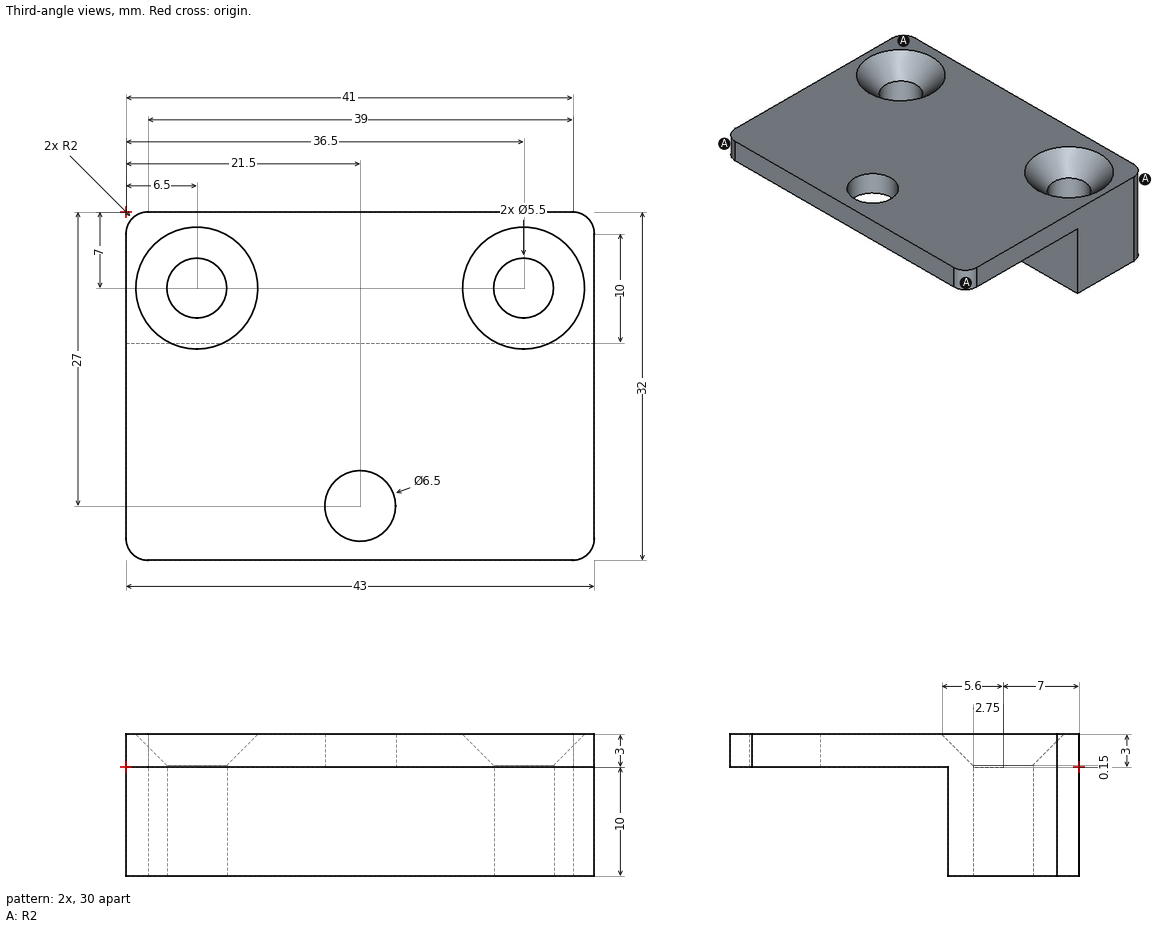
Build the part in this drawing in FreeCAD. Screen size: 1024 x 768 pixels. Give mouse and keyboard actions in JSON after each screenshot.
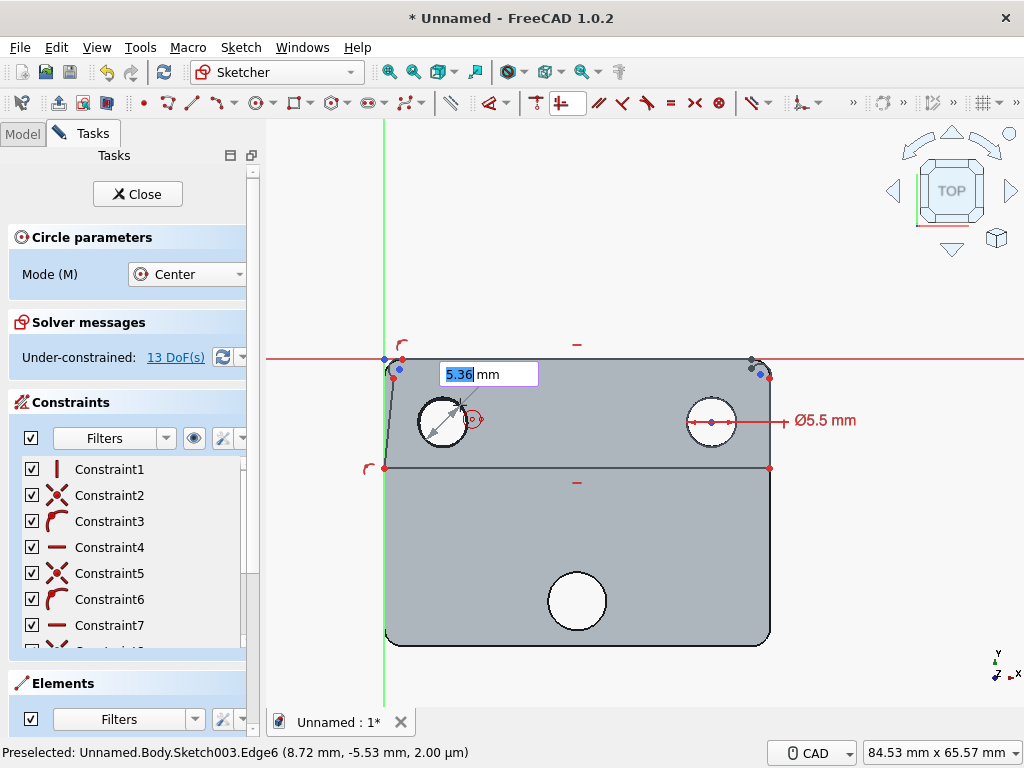
{"action": "type", "text": "5.5"}
{"action": "key", "text": "Return"}
{"action": "key", "text": "Escape"}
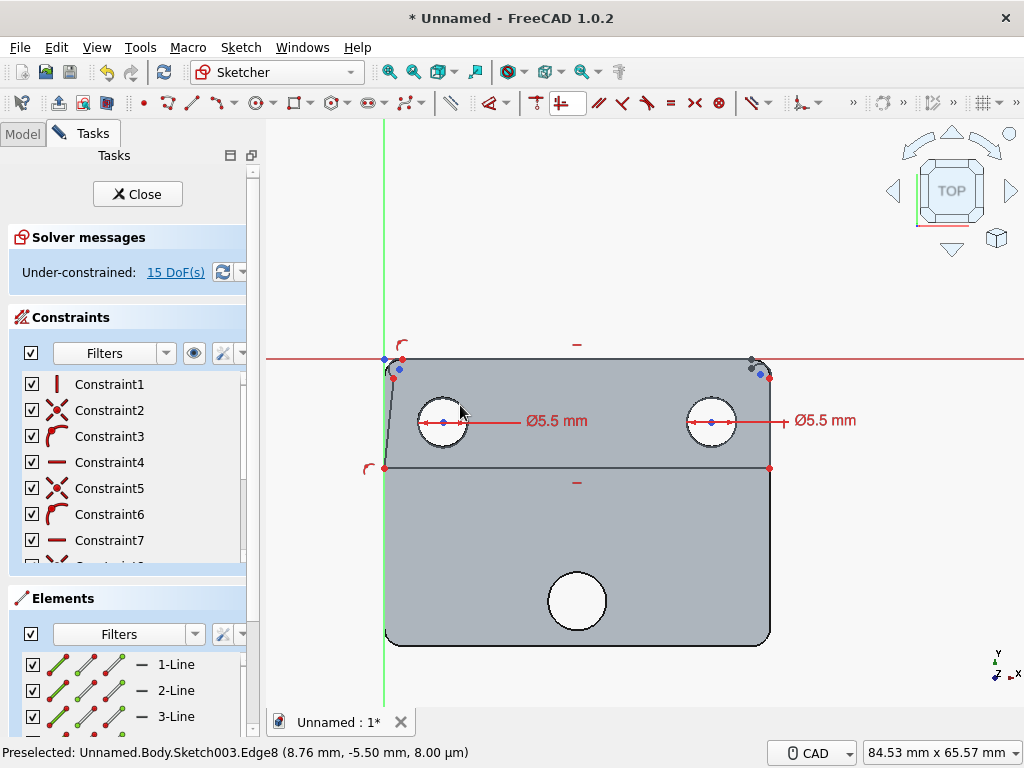
{"action": "left_click", "coordinate": [770, 405]}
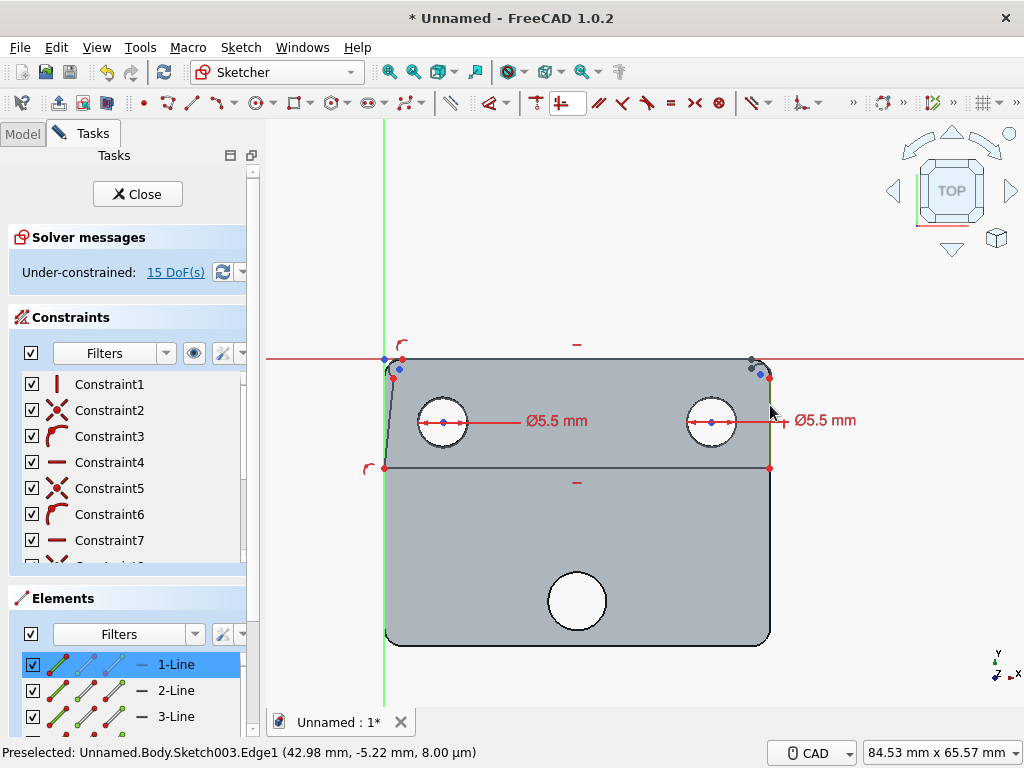
{"action": "scroll", "coordinate": [770, 369], "scroll_direction": "up", "scroll_amount": 3}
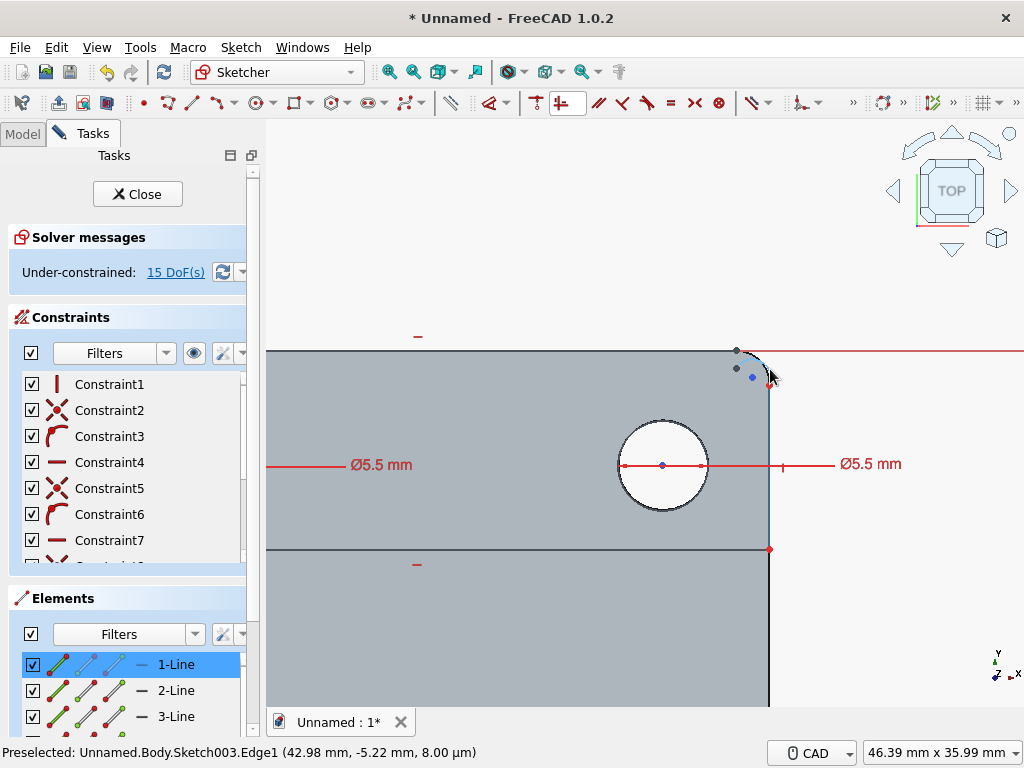
{"action": "left_click", "coordinate": [769, 369]}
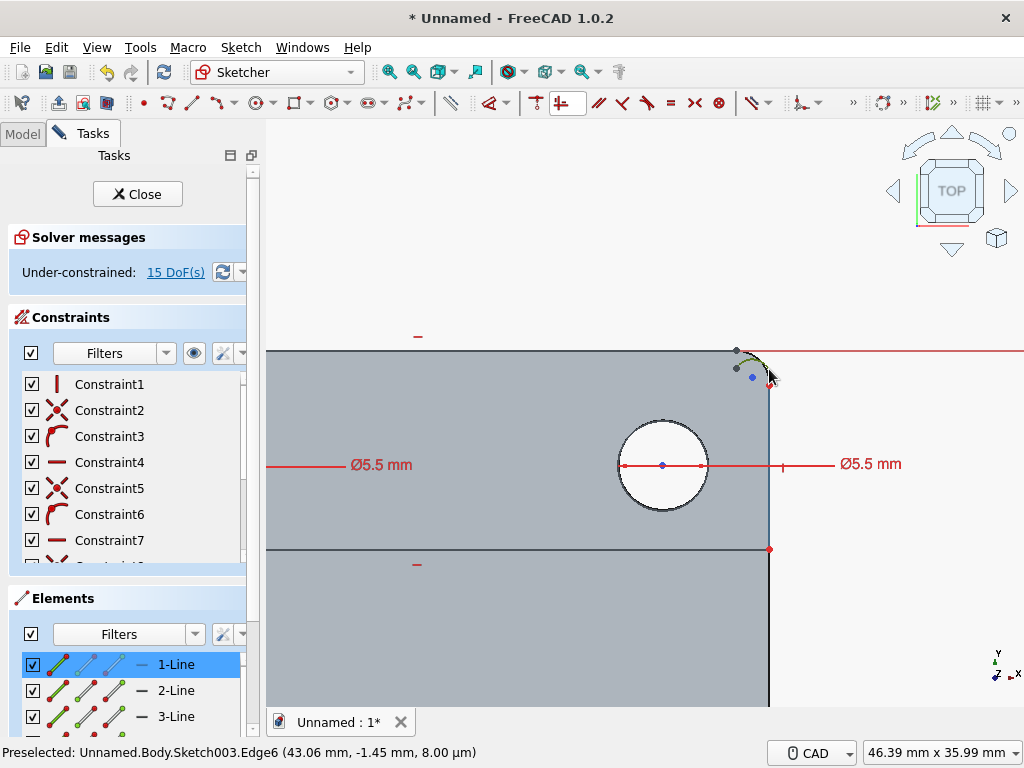
{"action": "key", "text": "t"}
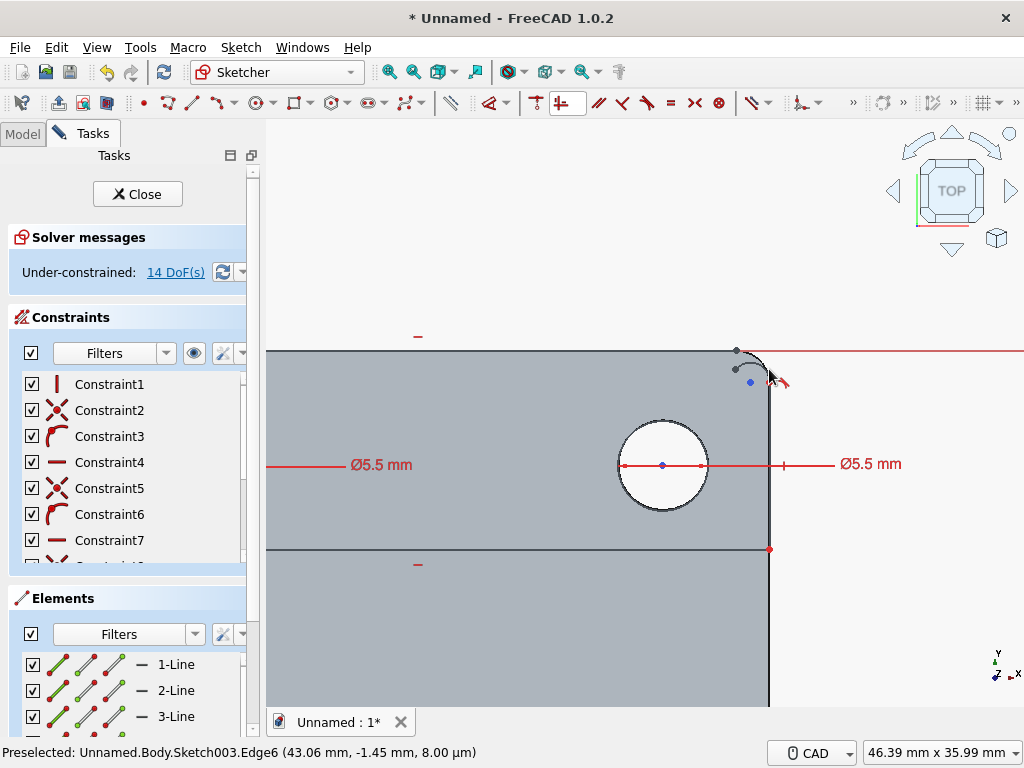
{"action": "scroll", "coordinate": [769, 369], "scroll_direction": "down", "scroll_amount": 3}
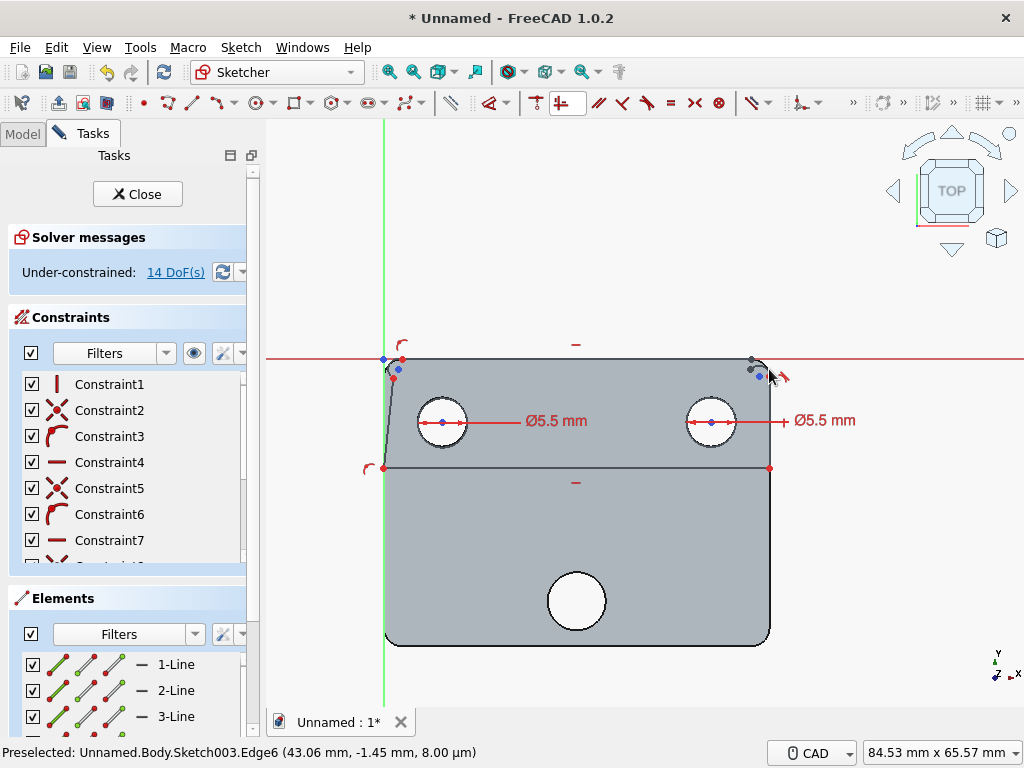
{"action": "scroll", "coordinate": [391, 405], "scroll_direction": "up", "scroll_amount": 4}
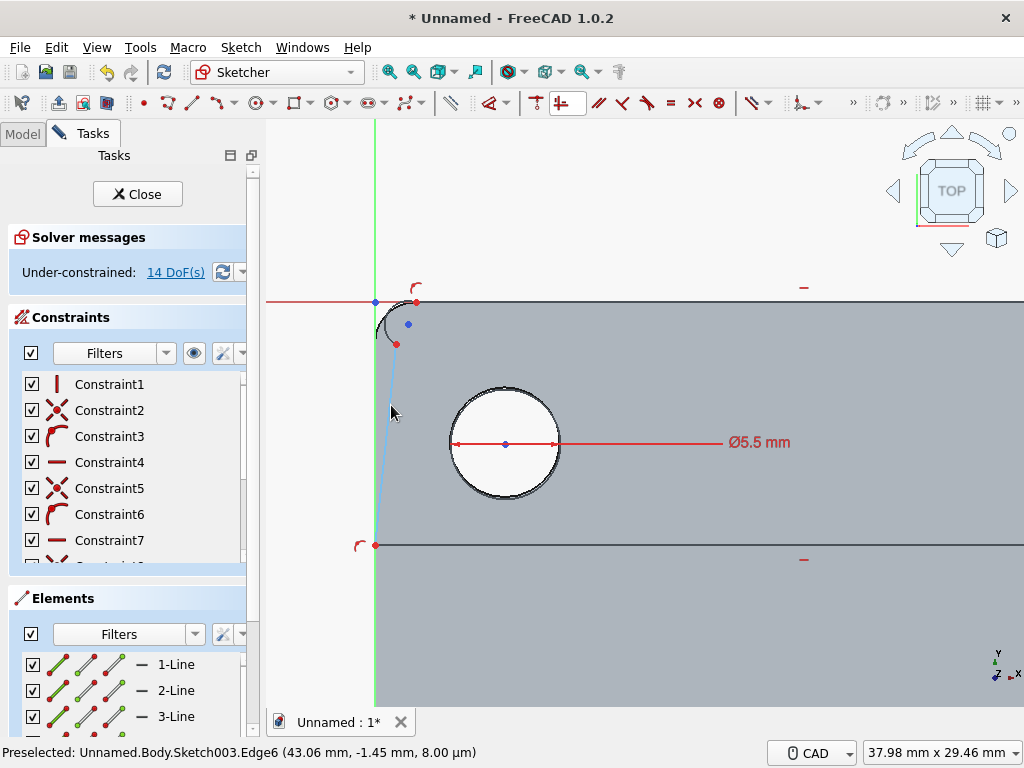
{"action": "left_click", "coordinate": [390, 405]}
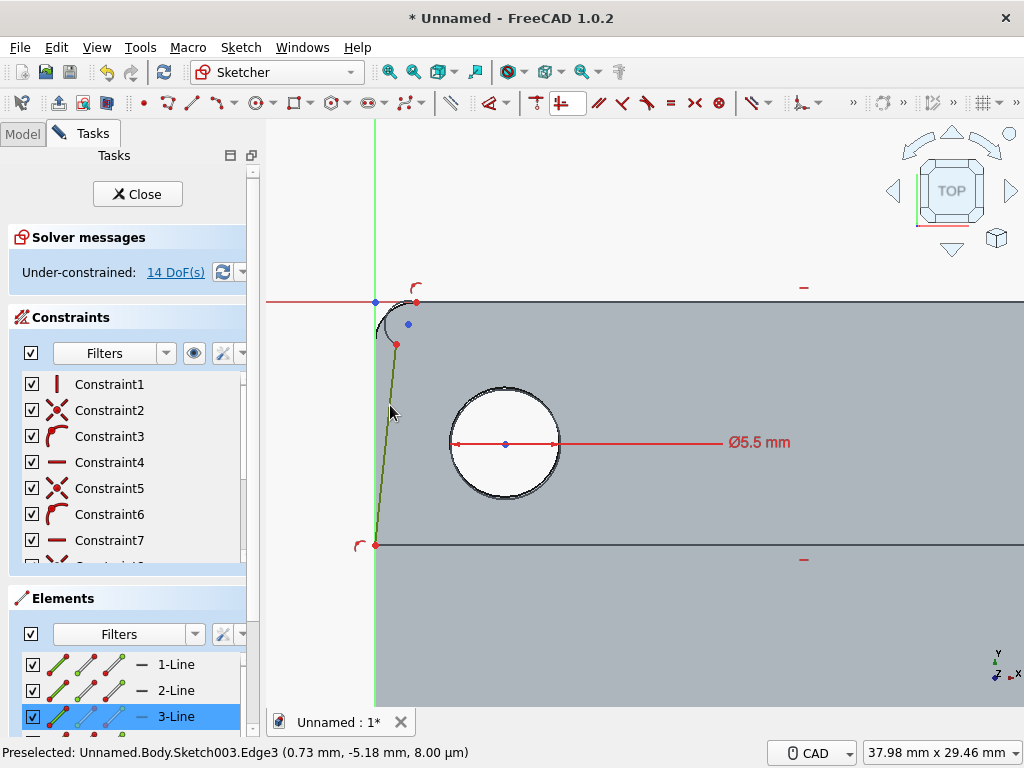
{"action": "left_click", "coordinate": [396, 305]}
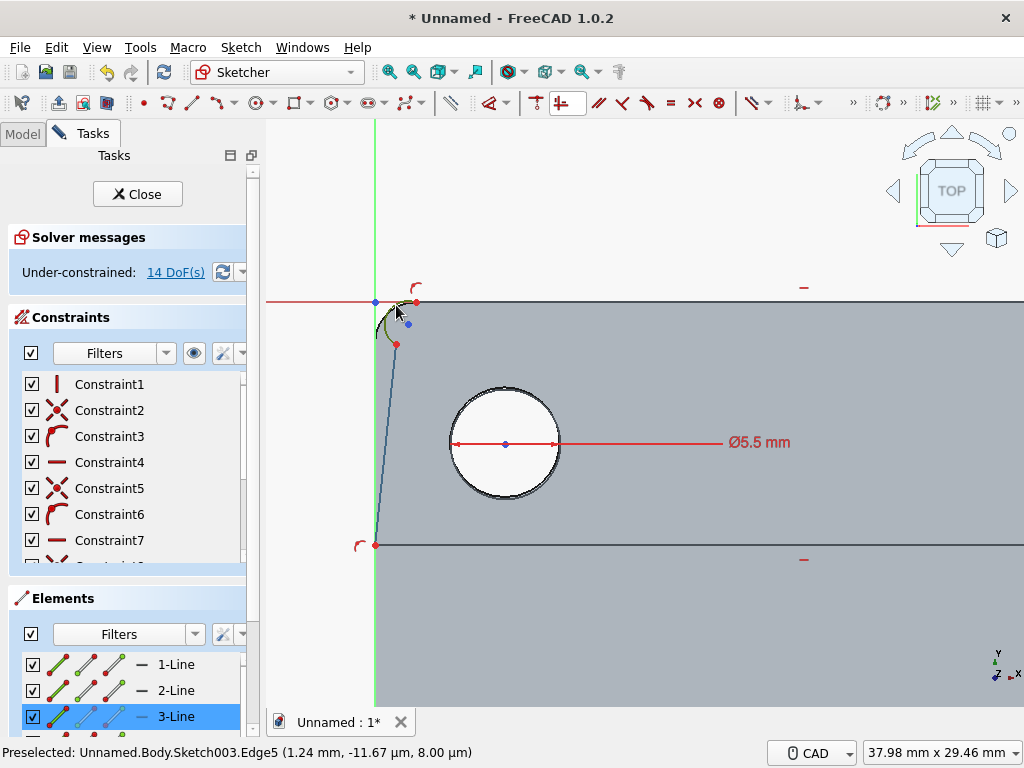
{"action": "key", "text": "t"}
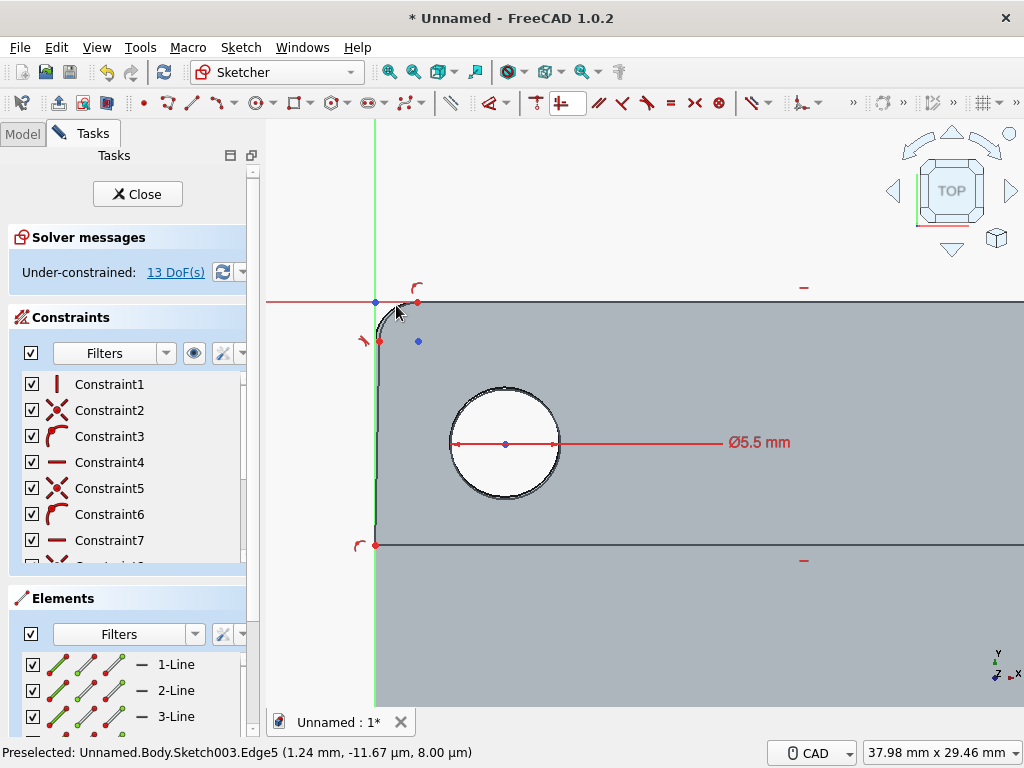
{"action": "left_click", "coordinate": [650, 302]}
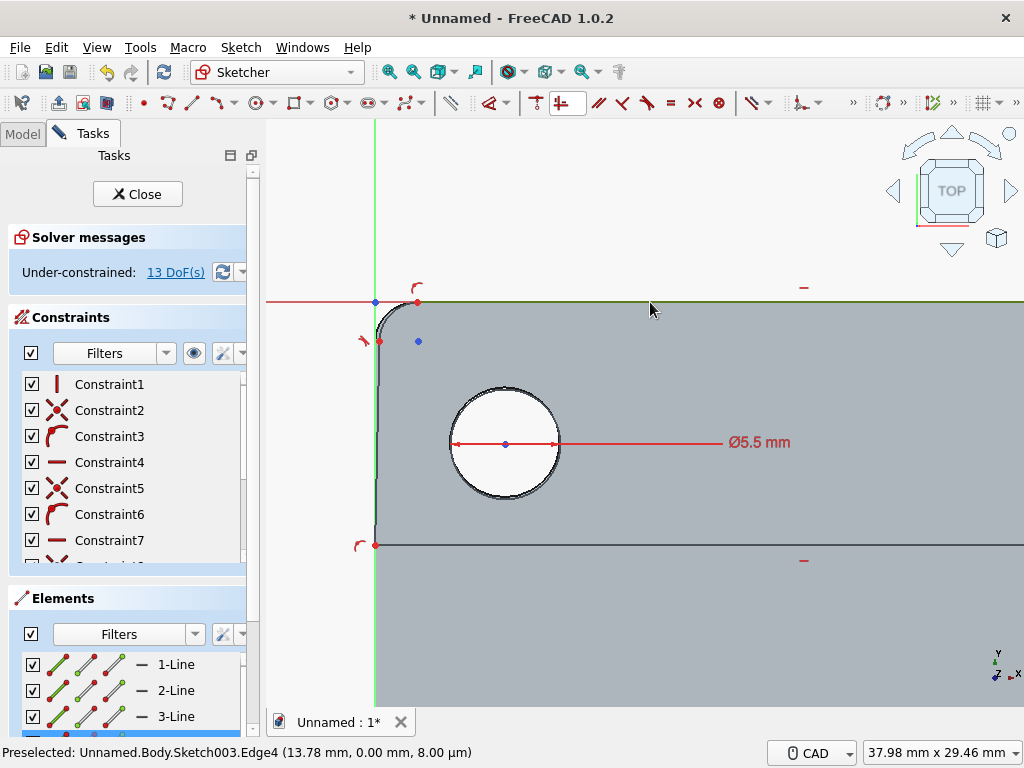
{"action": "left_click", "coordinate": [391, 314]}